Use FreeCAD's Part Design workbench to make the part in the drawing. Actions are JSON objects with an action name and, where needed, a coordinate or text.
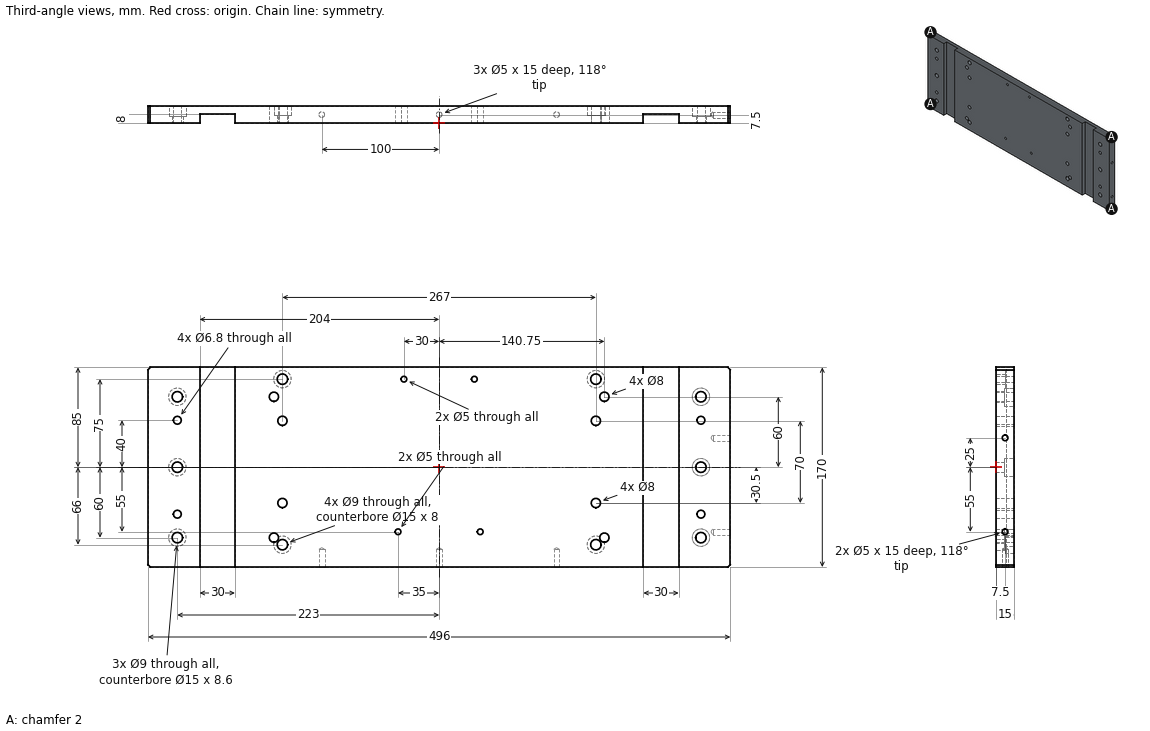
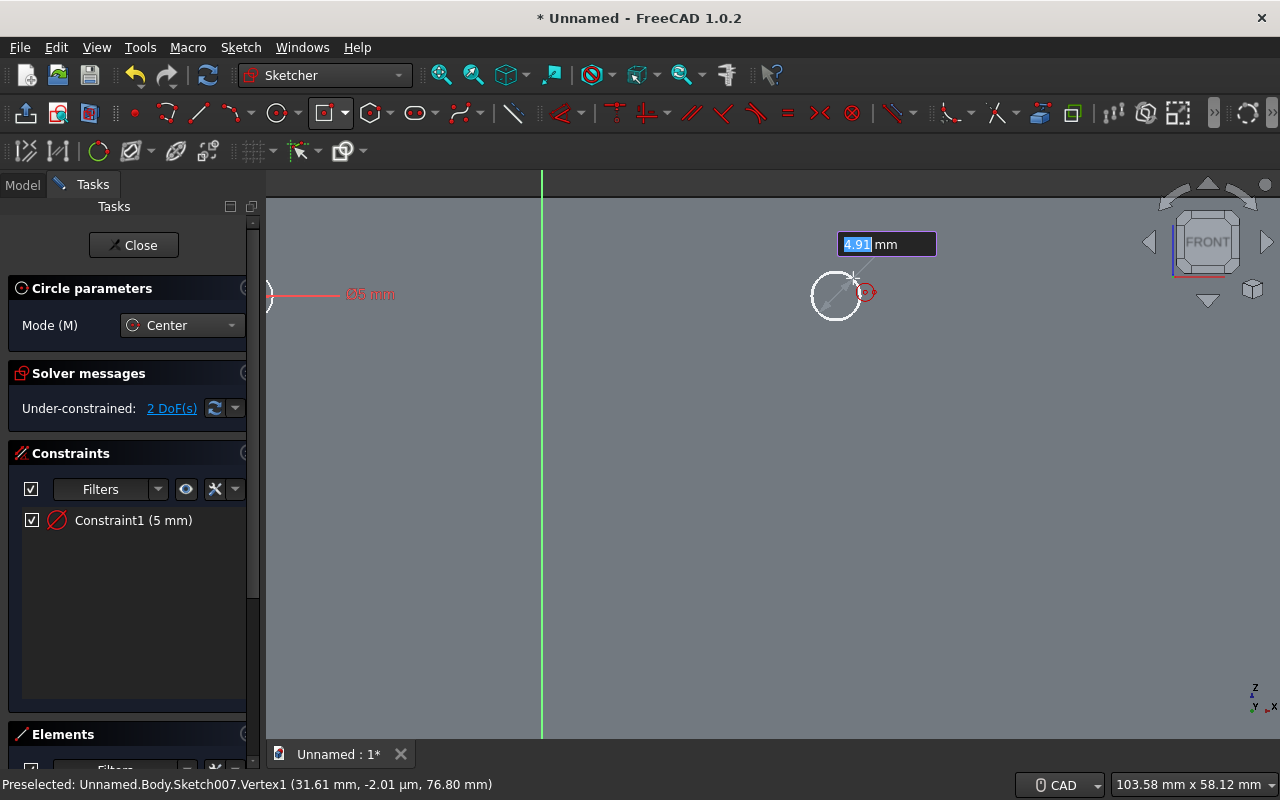
{"action": "type", "text": "5"}
{"action": "key", "text": "Return"}
{"action": "key", "text": "Escape"}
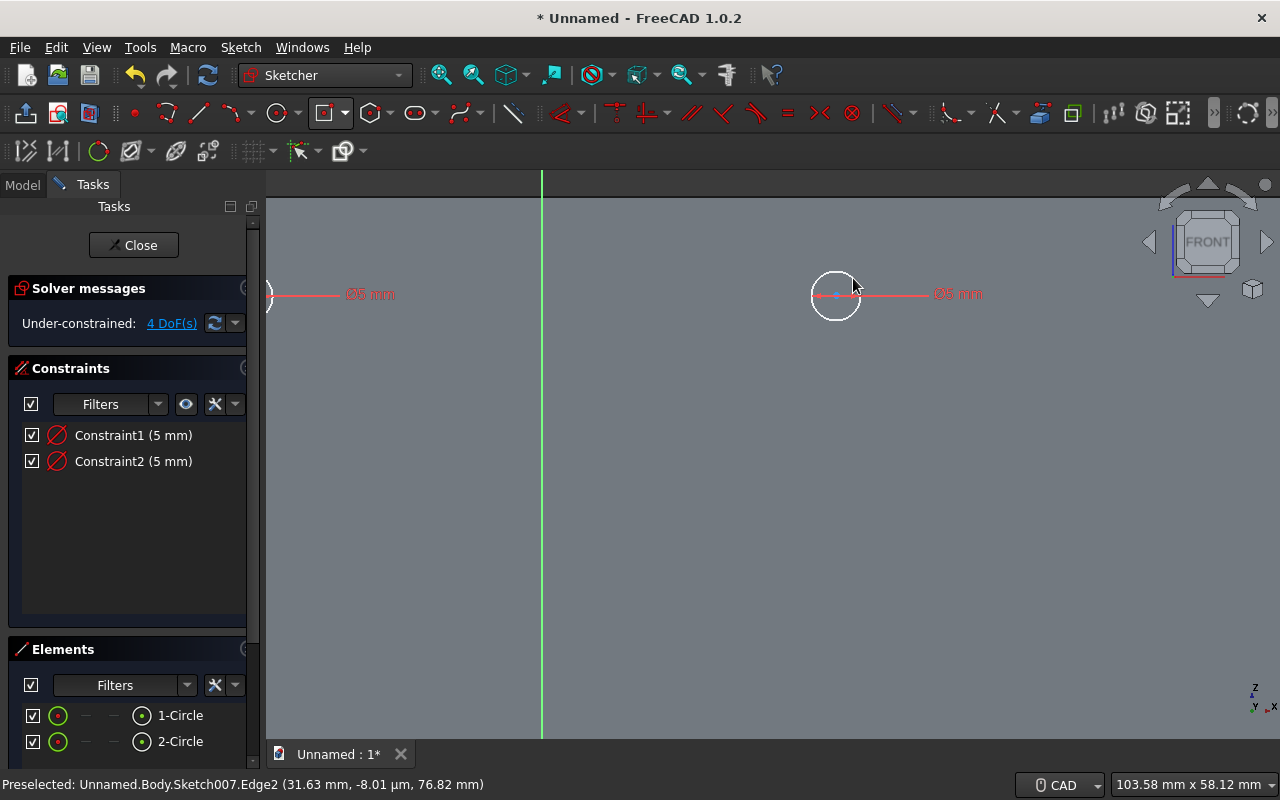
{"action": "scroll", "coordinate": [837, 295], "scroll_direction": "down", "scroll_amount": 4}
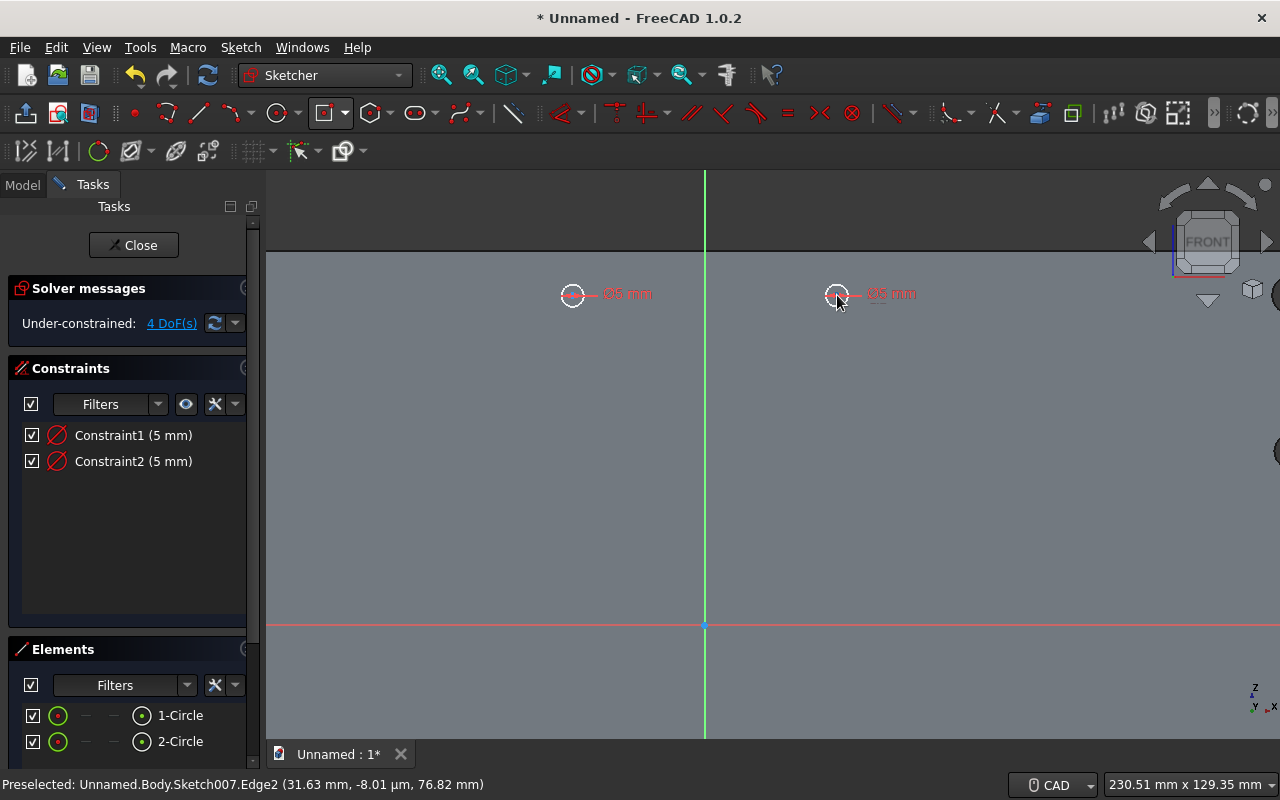
{"action": "left_click", "coordinate": [573, 296]}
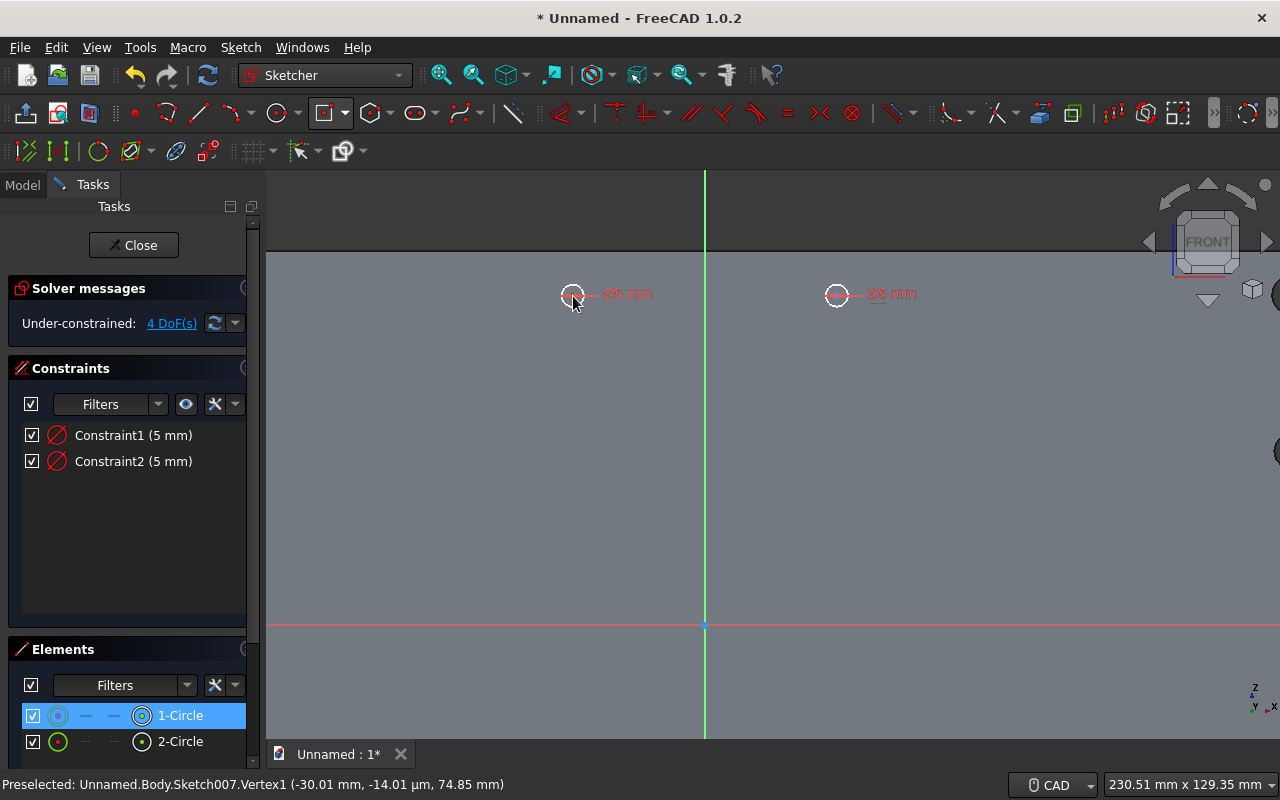
{"action": "left_click", "coordinate": [837, 296]}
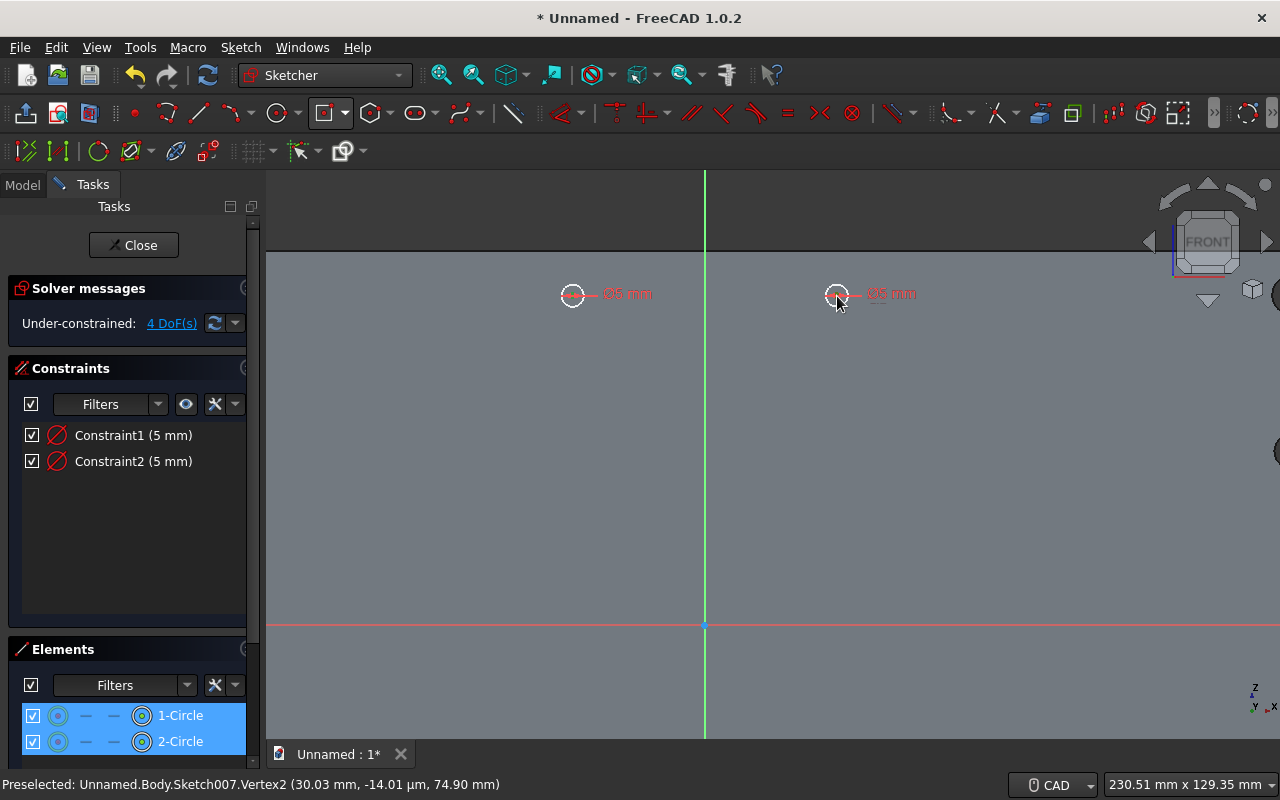
{"action": "left_click", "coordinate": [705, 674]}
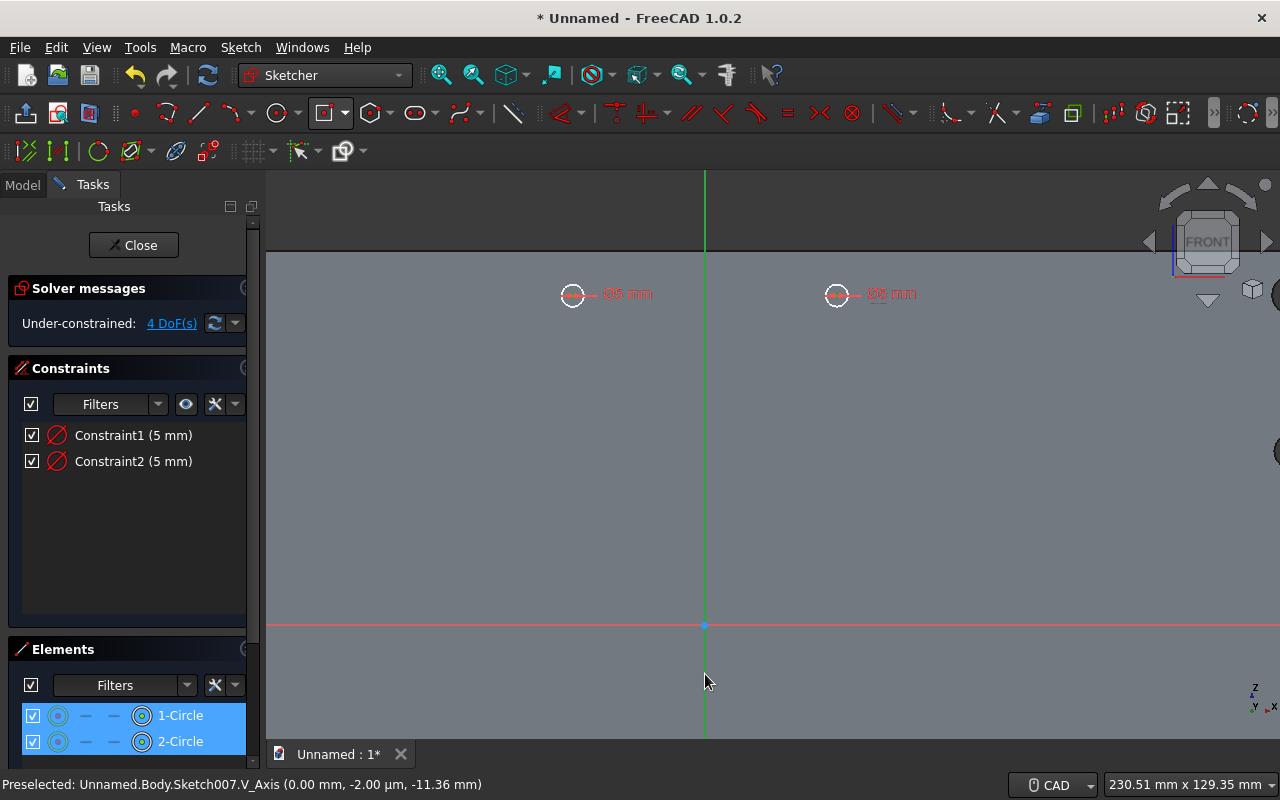
{"action": "left_click", "coordinate": [820, 114]}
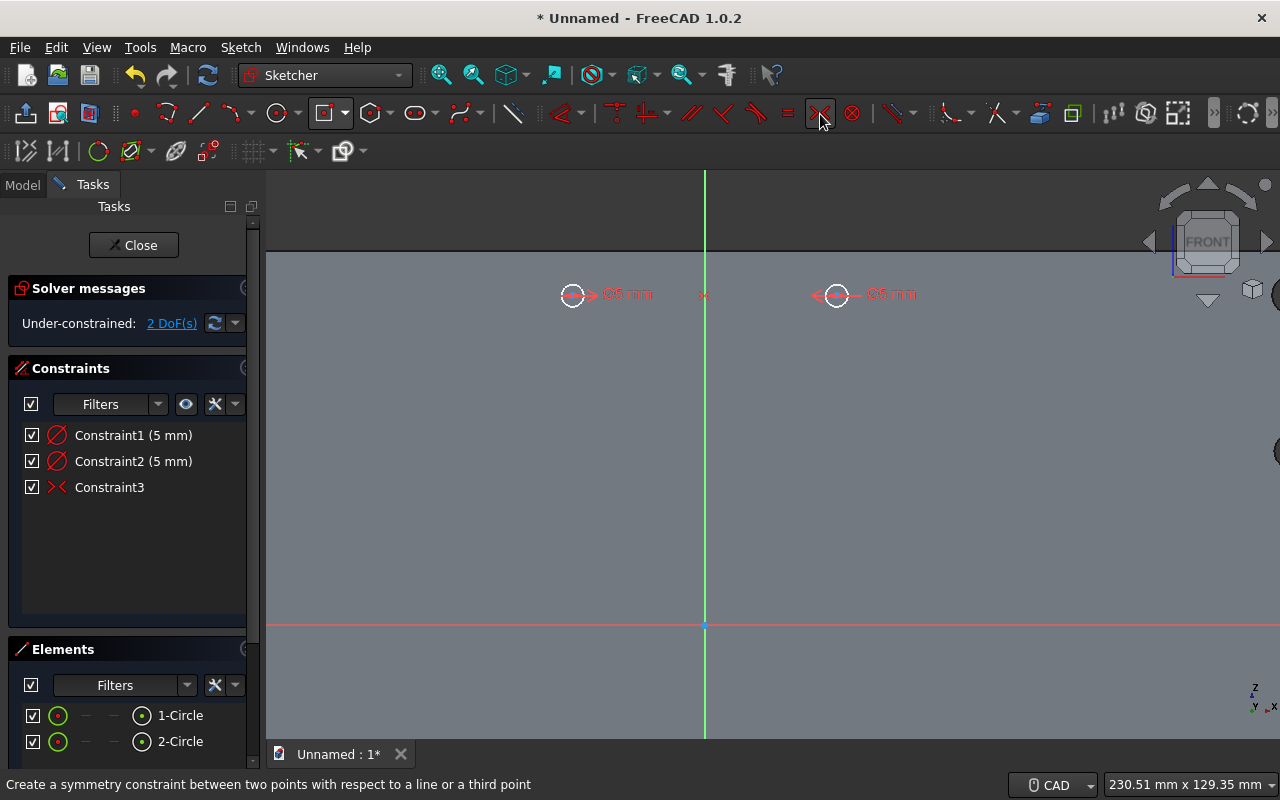
{"action": "left_click", "coordinate": [560, 114]}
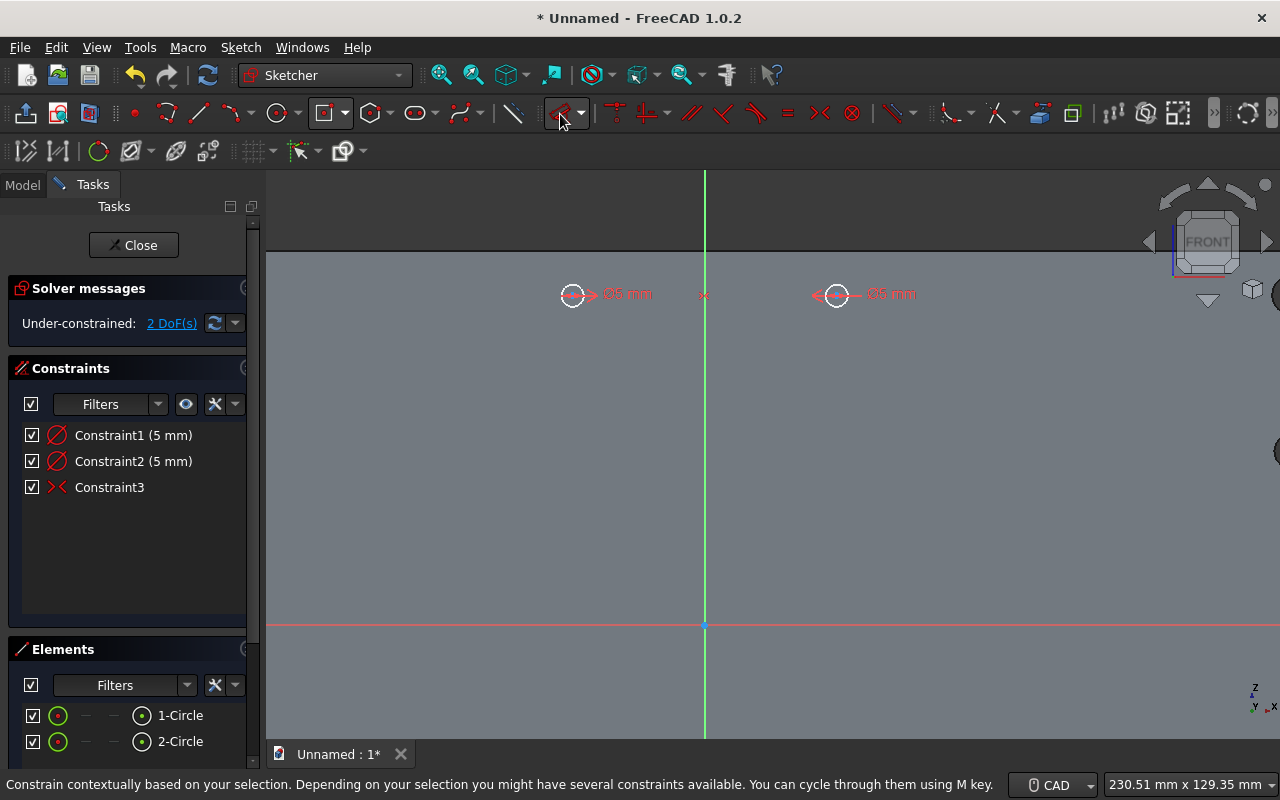
{"action": "left_click", "coordinate": [573, 296]}
{"action": "left_click", "coordinate": [639, 659]}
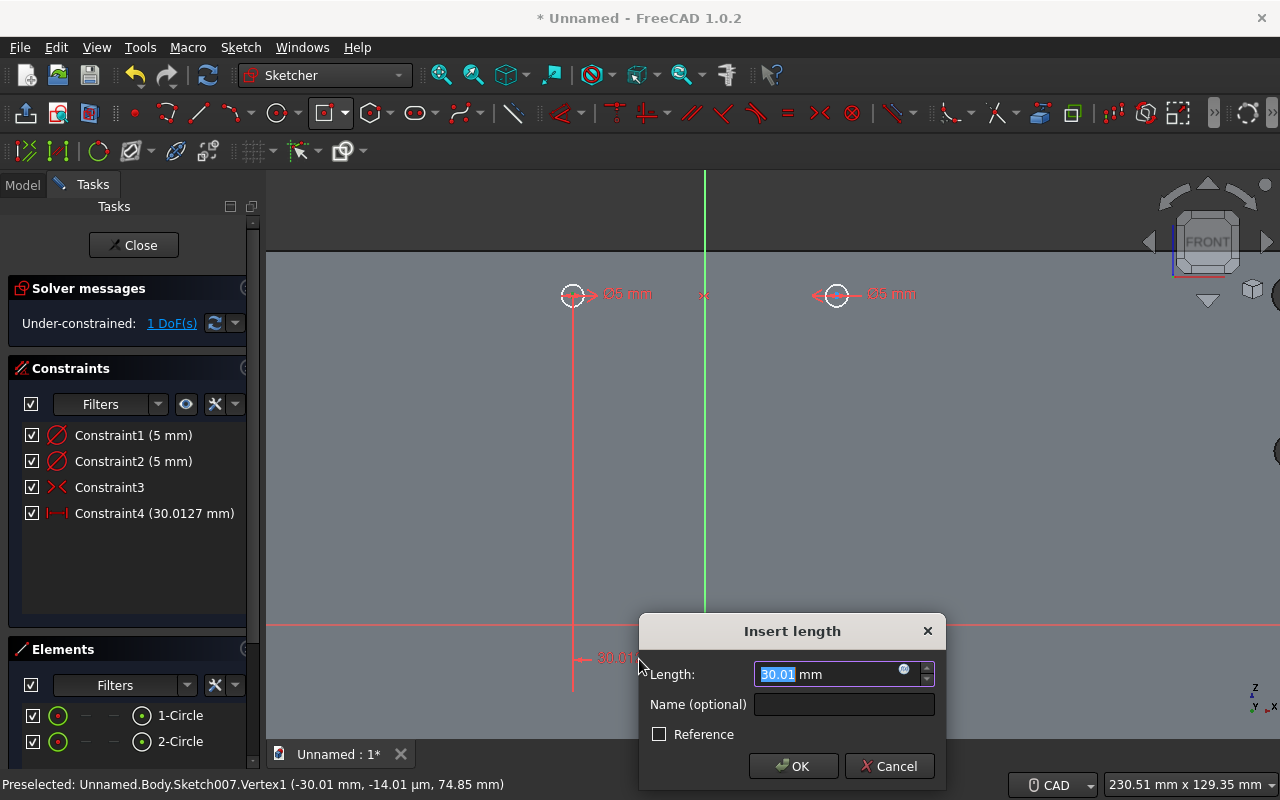
{"action": "type", "text": "30"}
{"action": "key", "text": "Return"}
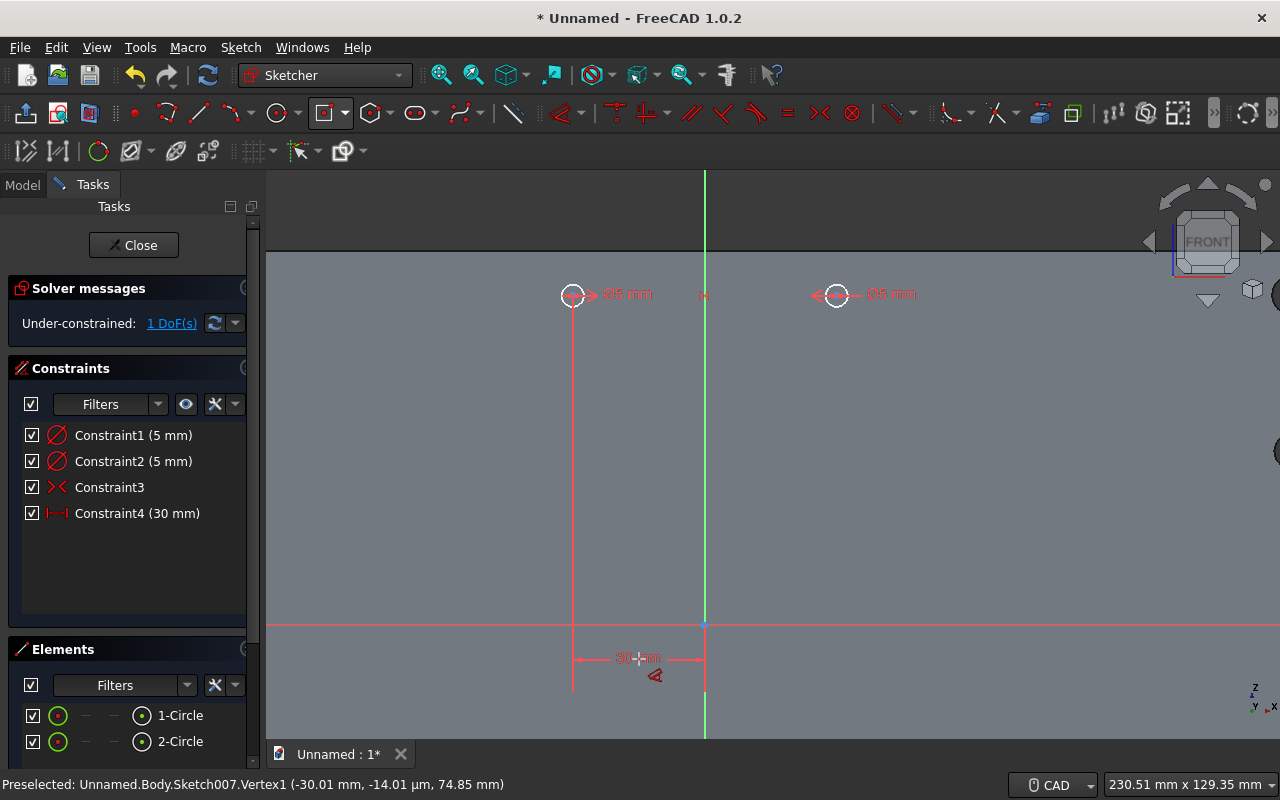
{"action": "left_click", "coordinate": [573, 296]}
{"action": "left_click", "coordinate": [539, 460]}